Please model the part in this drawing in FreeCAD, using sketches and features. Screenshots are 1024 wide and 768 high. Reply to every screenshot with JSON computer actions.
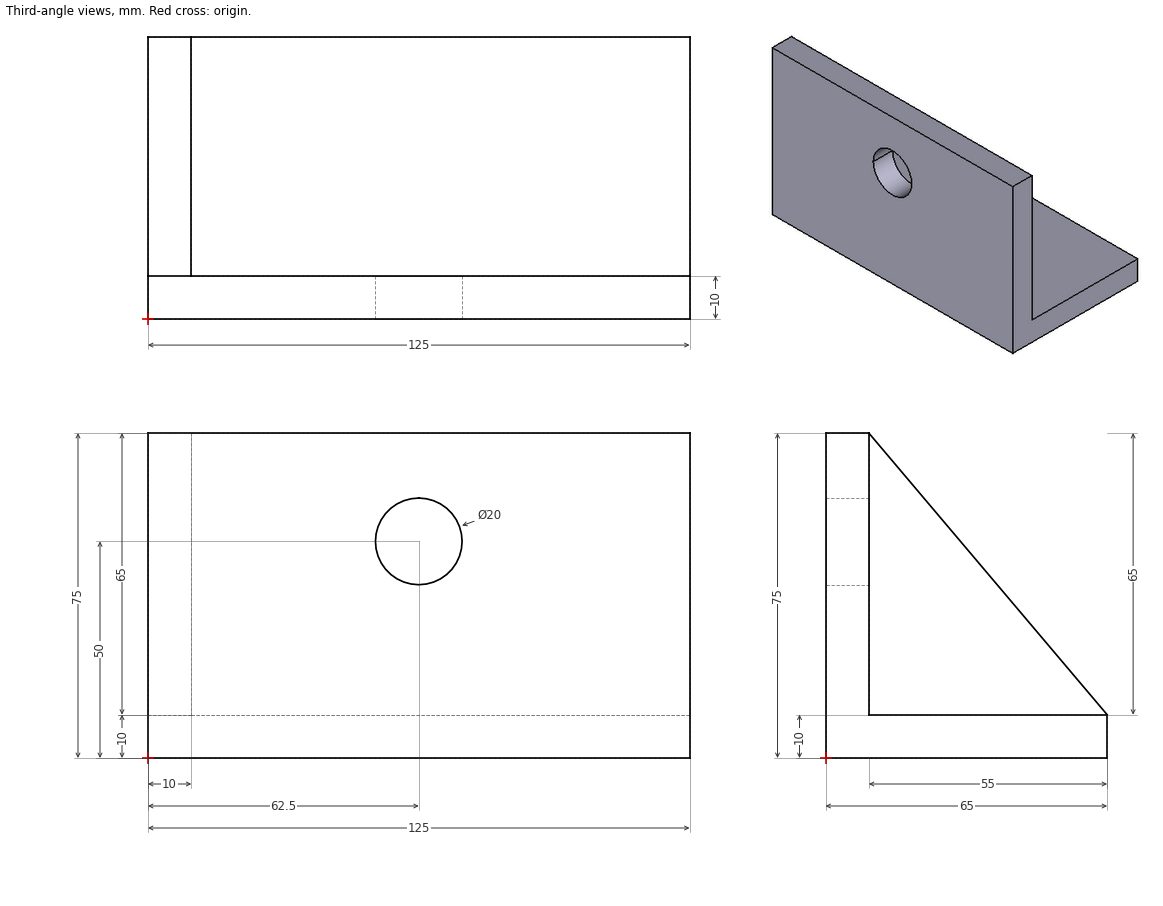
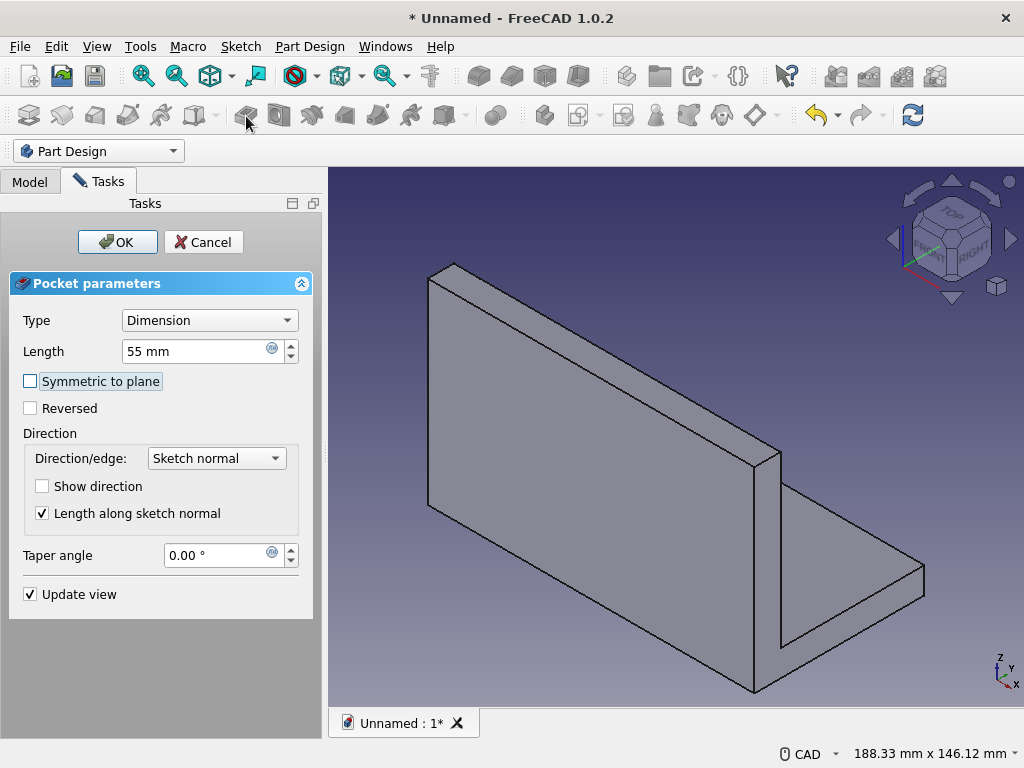
{"action": "left_click", "coordinate": [118, 242]}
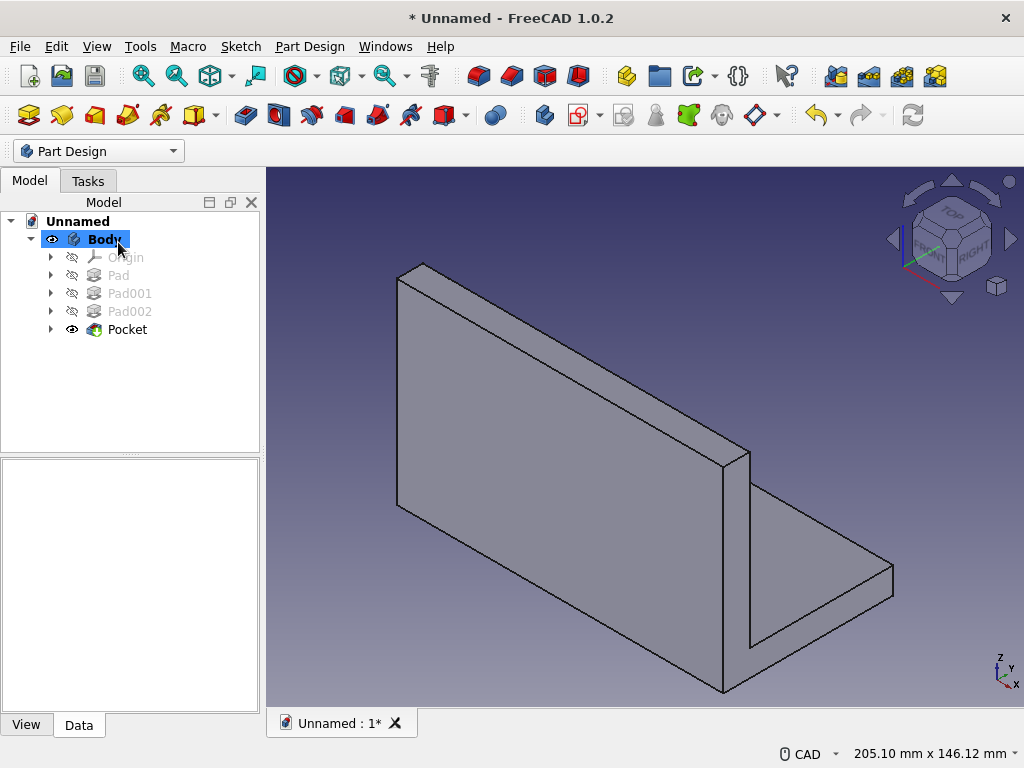
{"action": "key", "text": "4"}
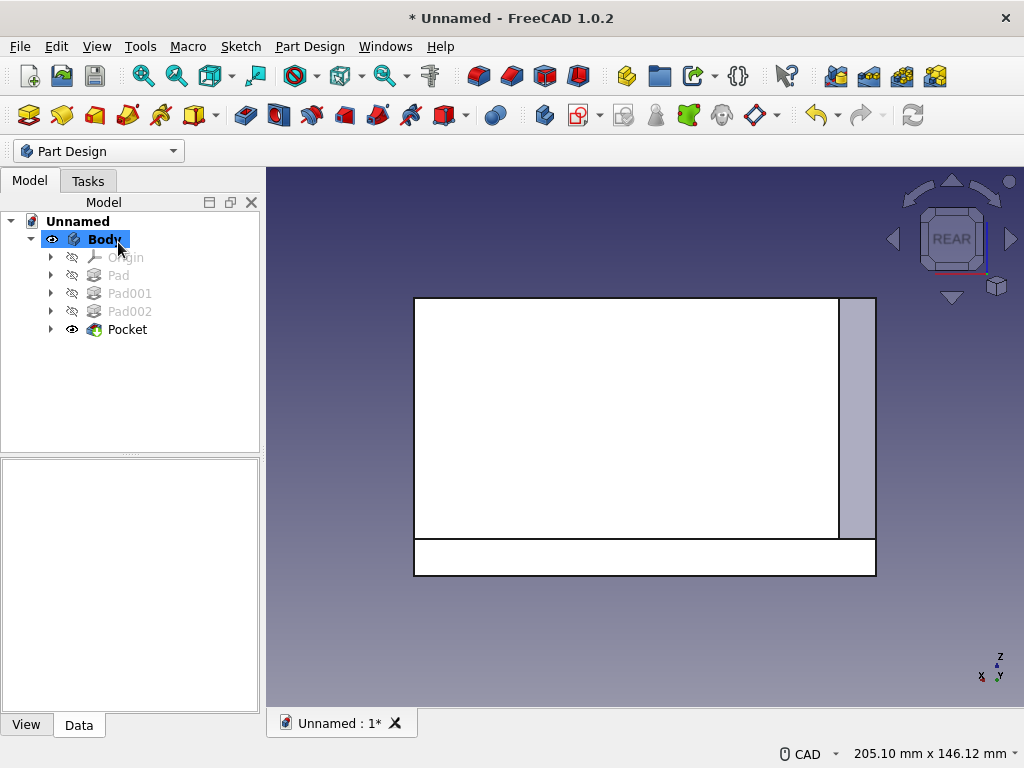
{"action": "left_click", "coordinate": [566, 418]}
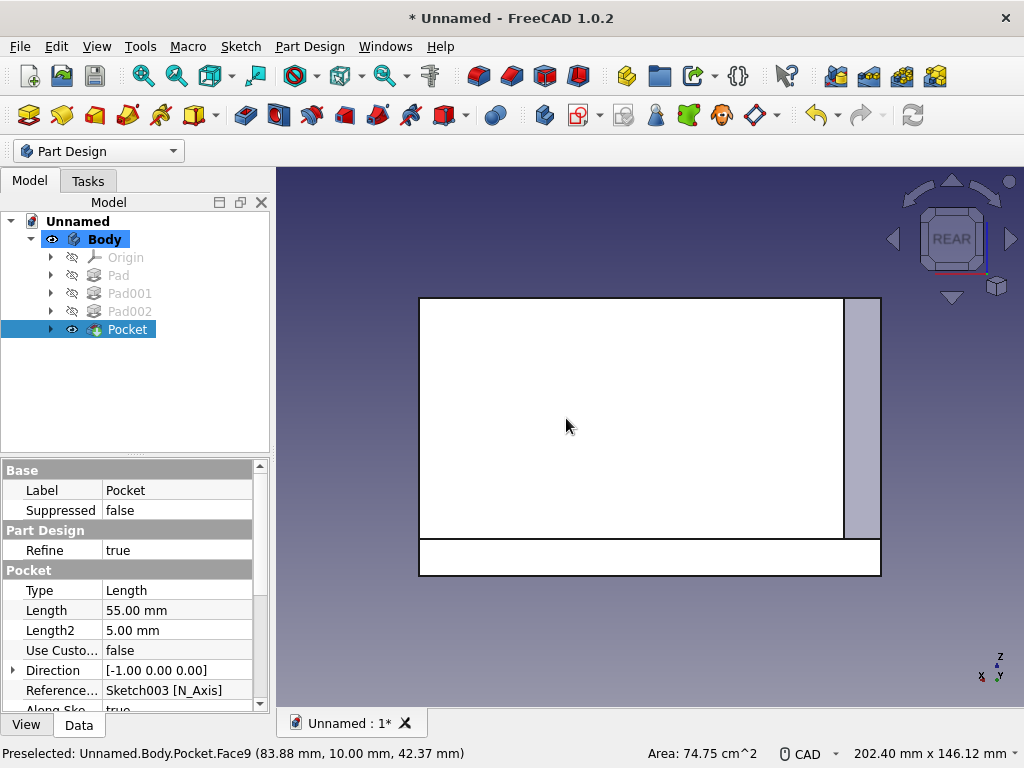
{"action": "left_click", "coordinate": [578, 116]}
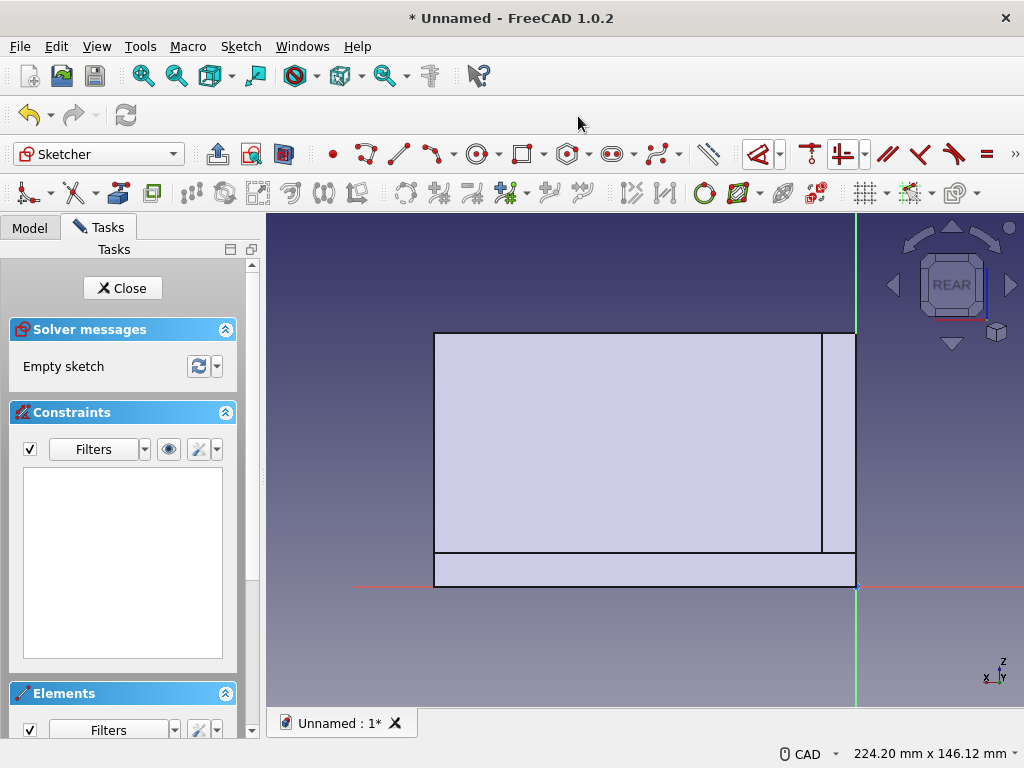
{"action": "left_click", "coordinate": [284, 154]}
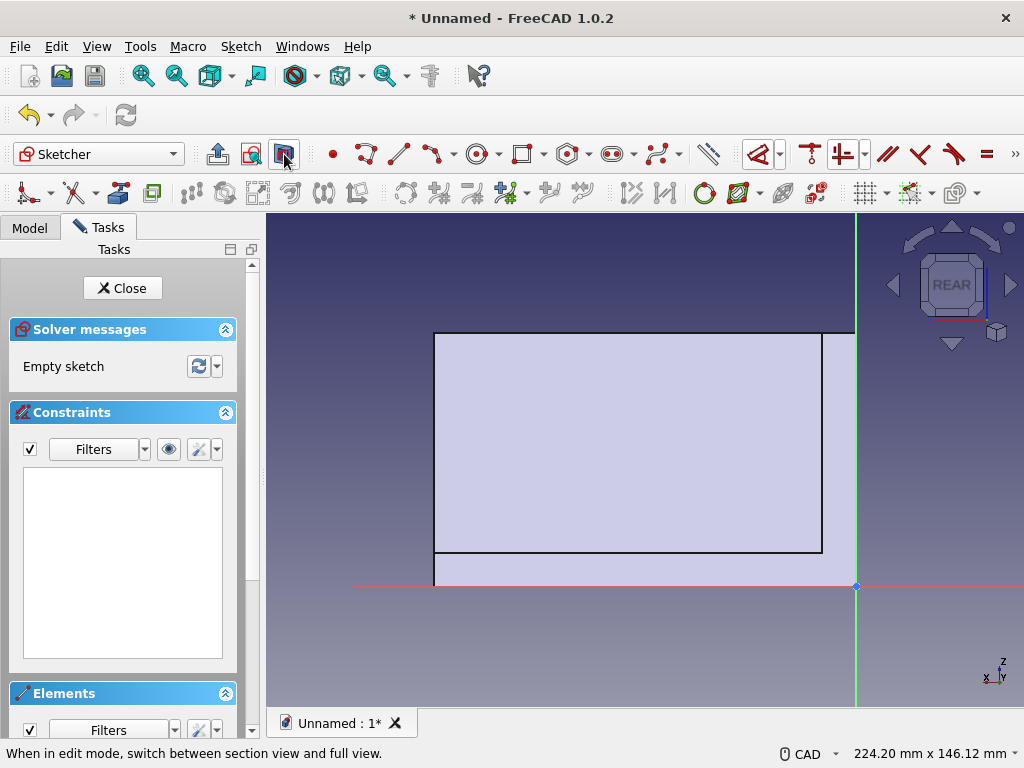
{"action": "scroll", "coordinate": [662, 407], "scroll_direction": "up", "scroll_amount": 8}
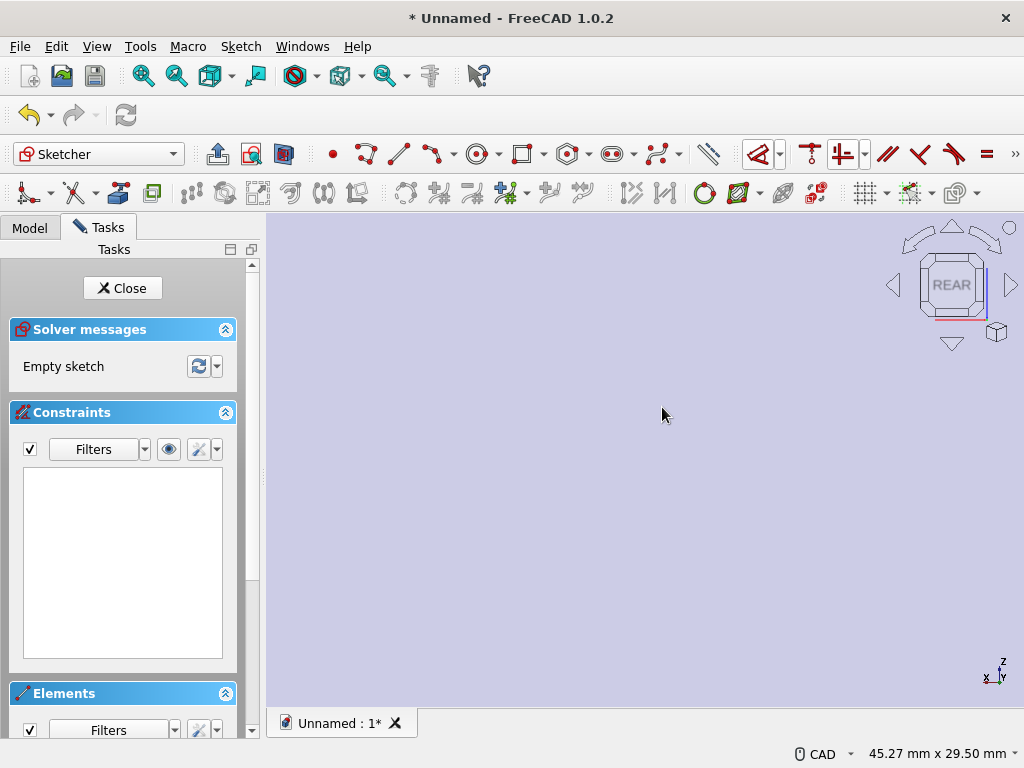
{"action": "left_click", "coordinate": [476, 154]}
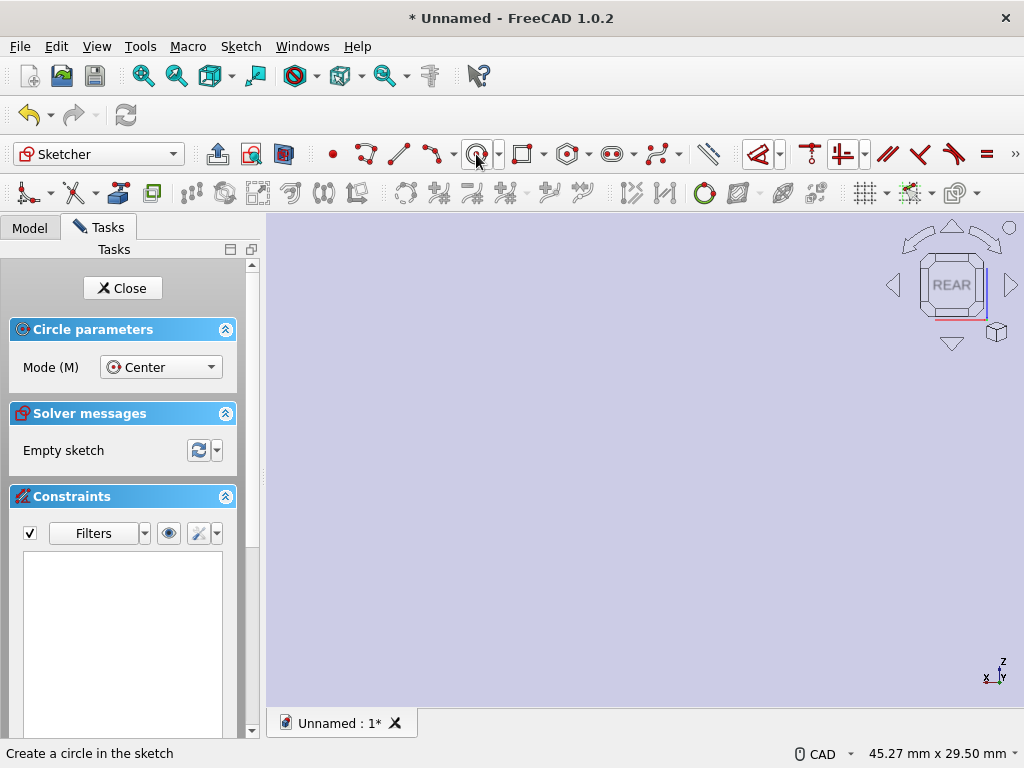
{"action": "left_click", "coordinate": [576, 459]}
{"action": "left_click", "coordinate": [694, 340]}
{"action": "key", "text": "Escape"}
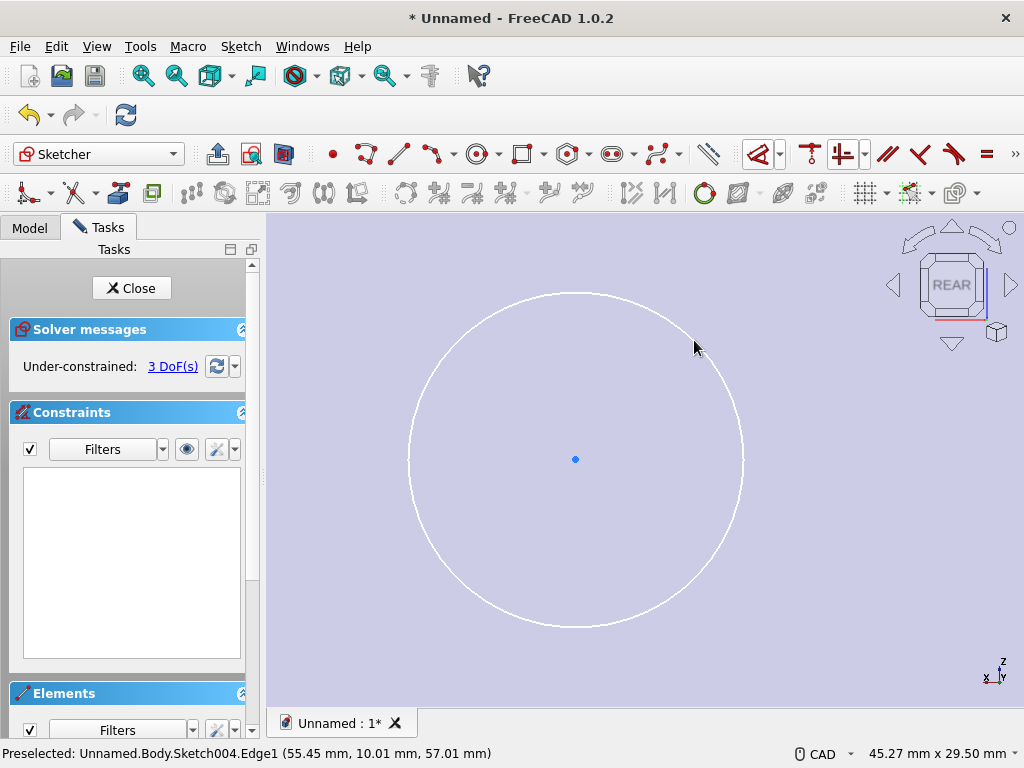
{"action": "left_click", "coordinate": [694, 341]}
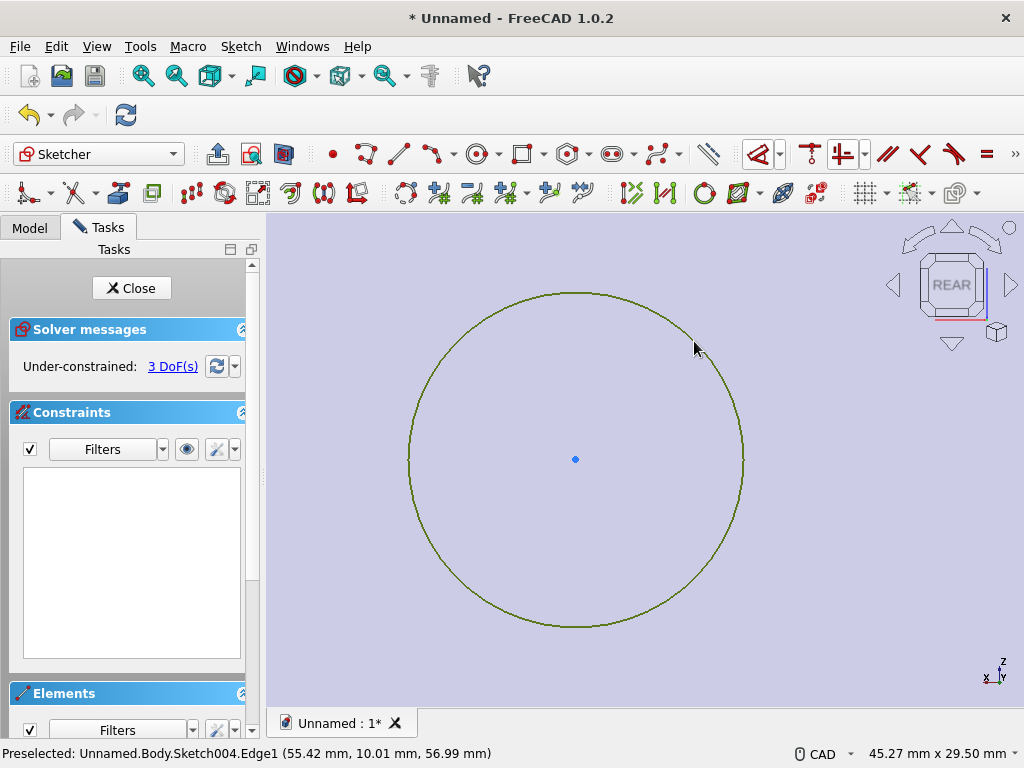
{"action": "key", "text": "k o"}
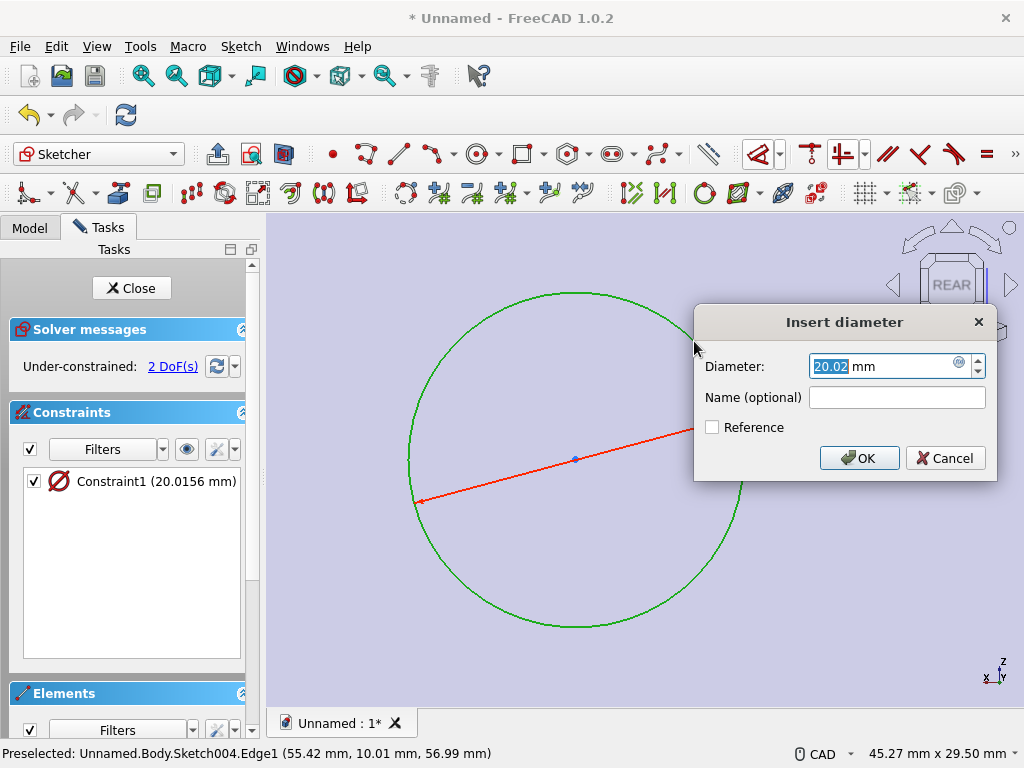
{"action": "type", "text": "20"}
{"action": "key", "text": "Return"}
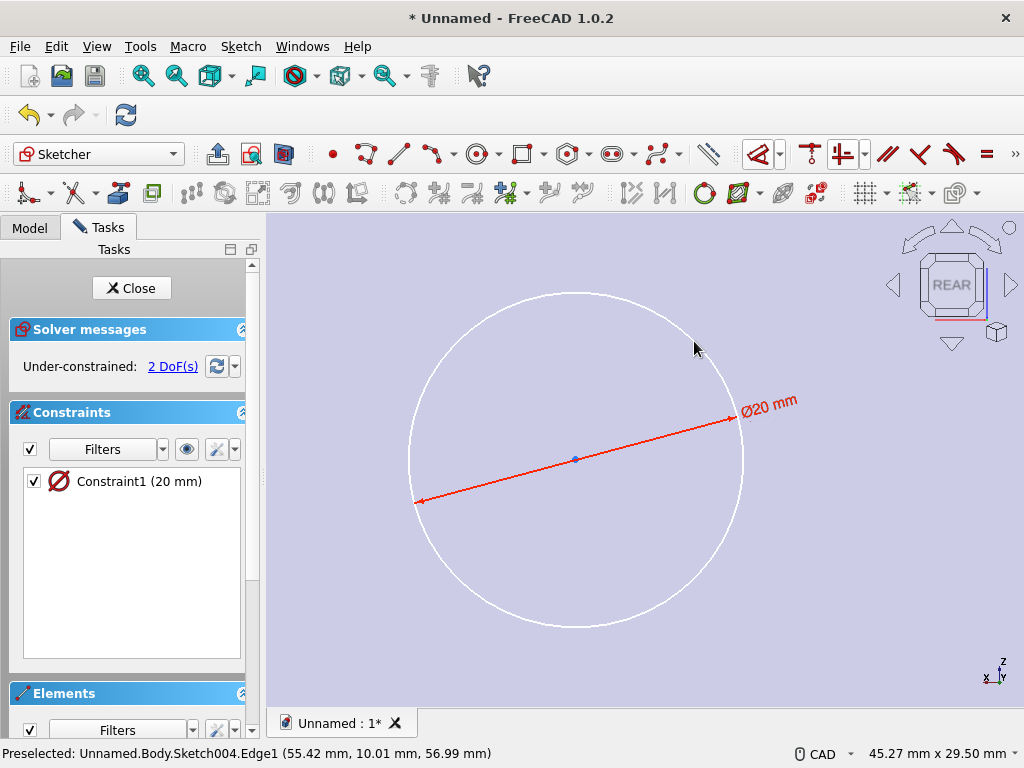
{"action": "left_click", "coordinate": [576, 460]}